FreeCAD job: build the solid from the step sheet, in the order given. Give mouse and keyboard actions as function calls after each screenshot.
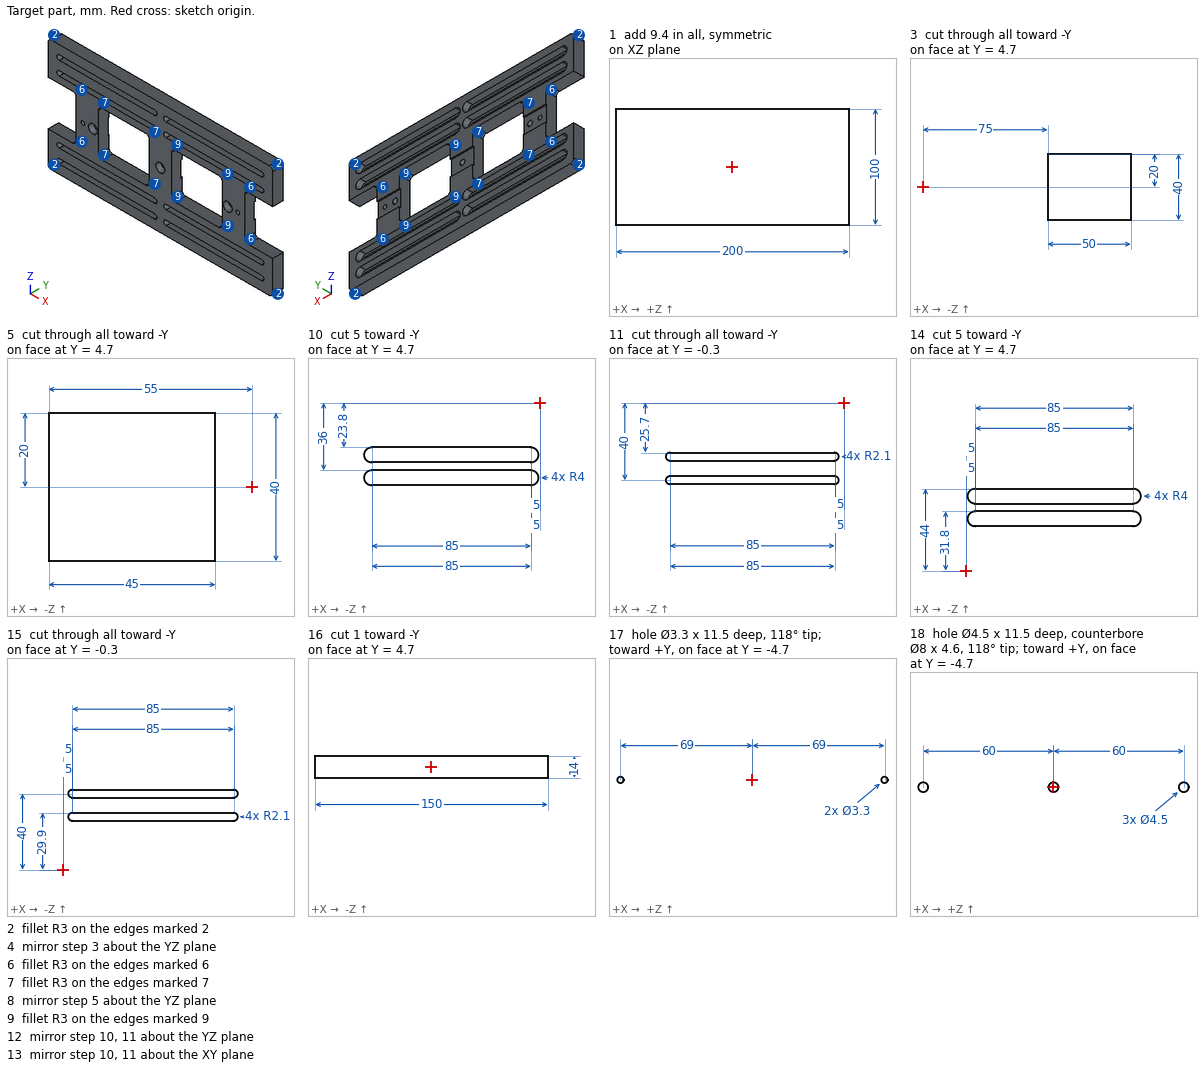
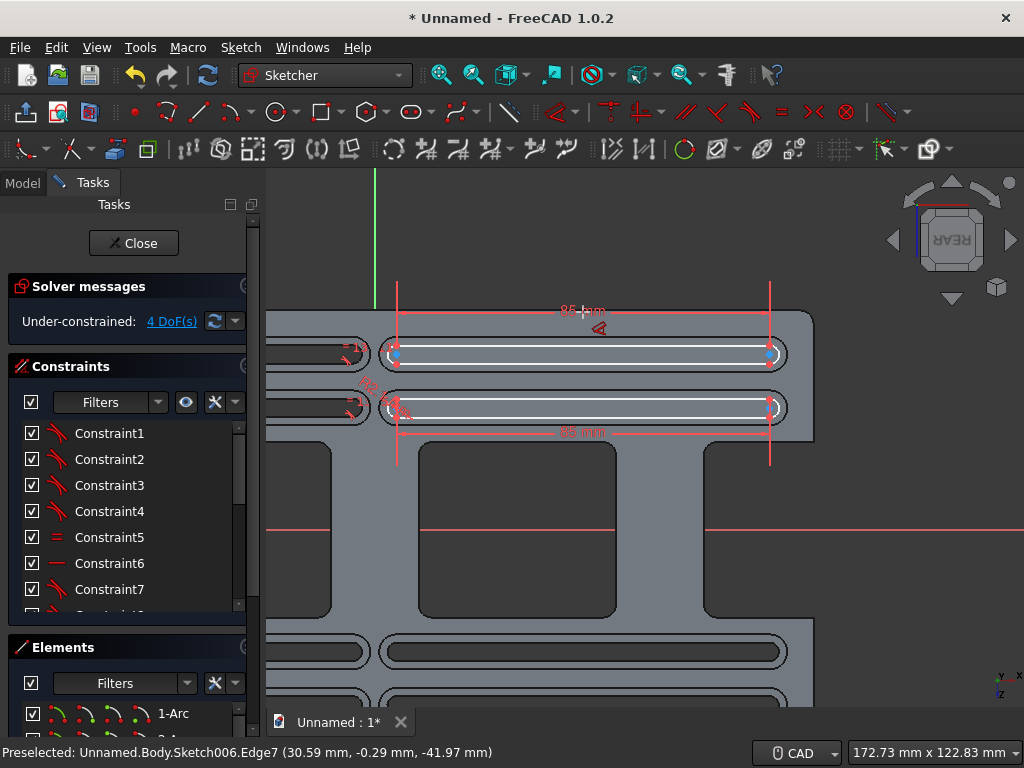
scroll(397, 399, up, 3)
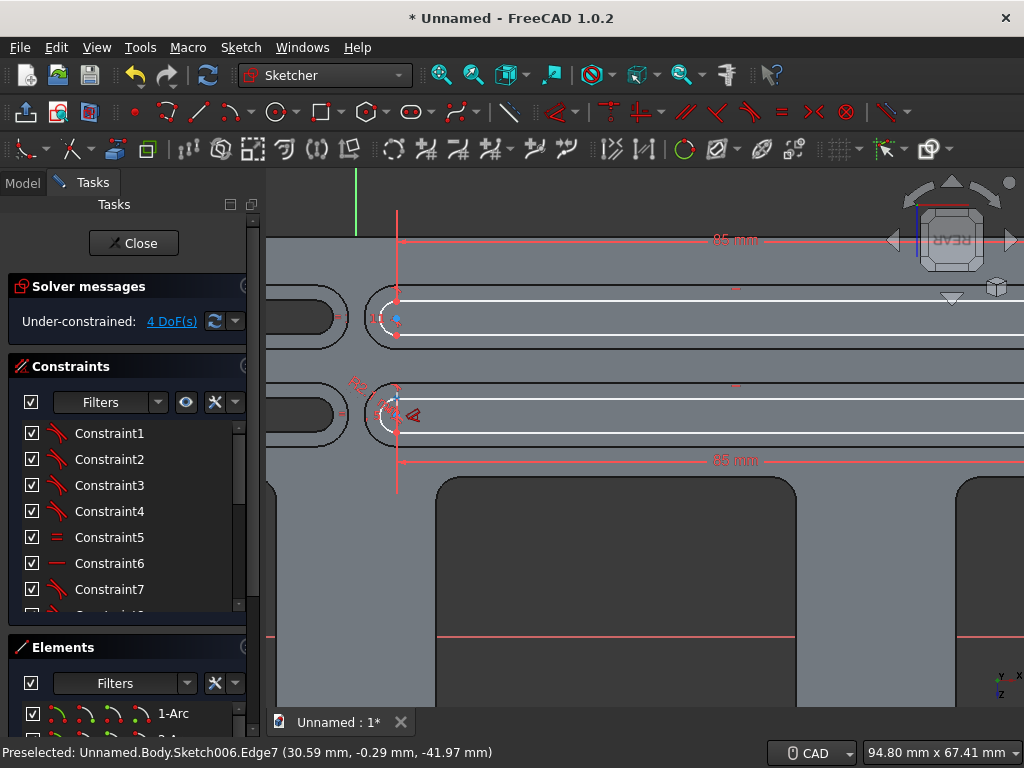
click(397, 399)
click(377, 671)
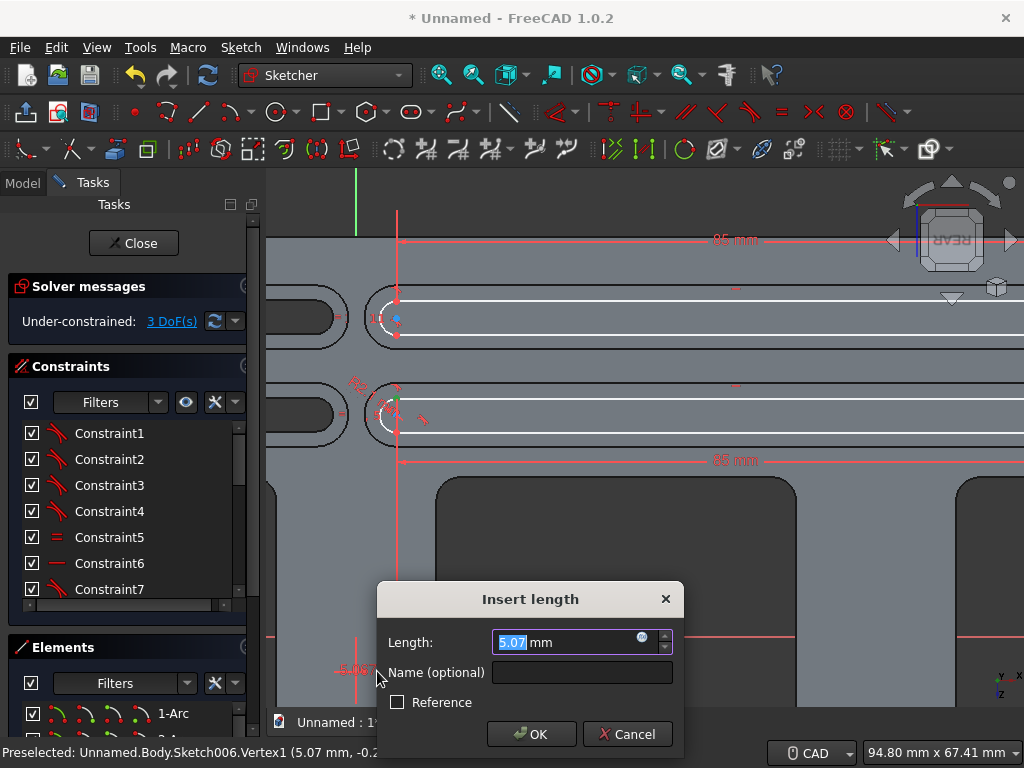
text(5)
key(Return)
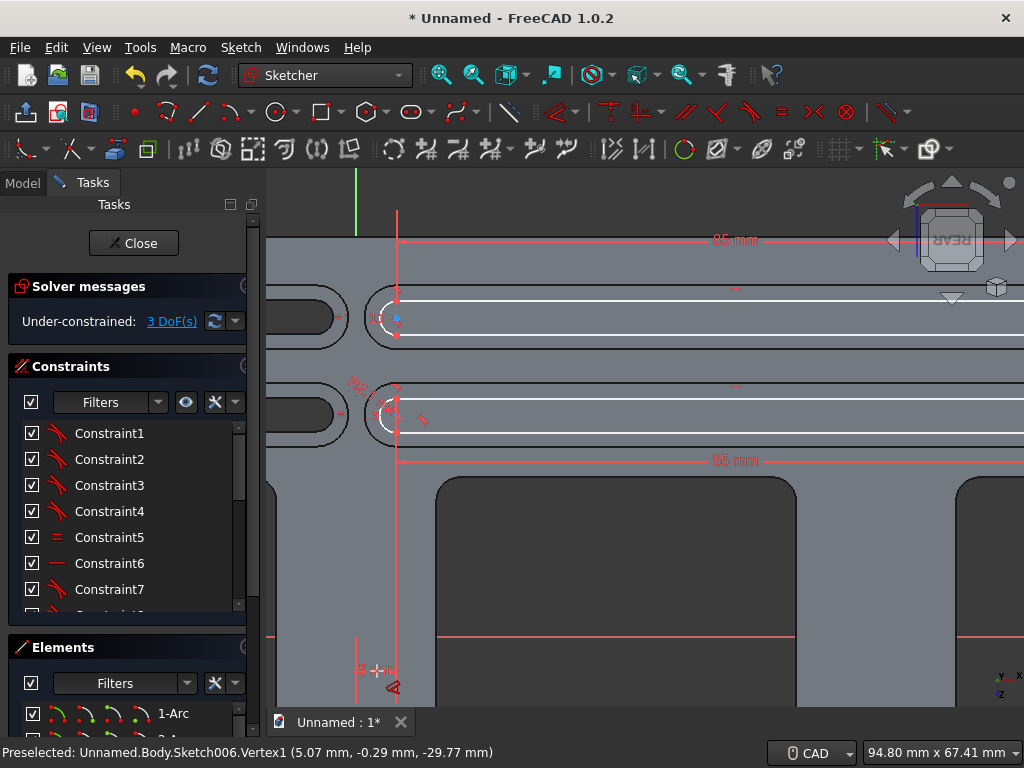
click(397, 301)
click(377, 267)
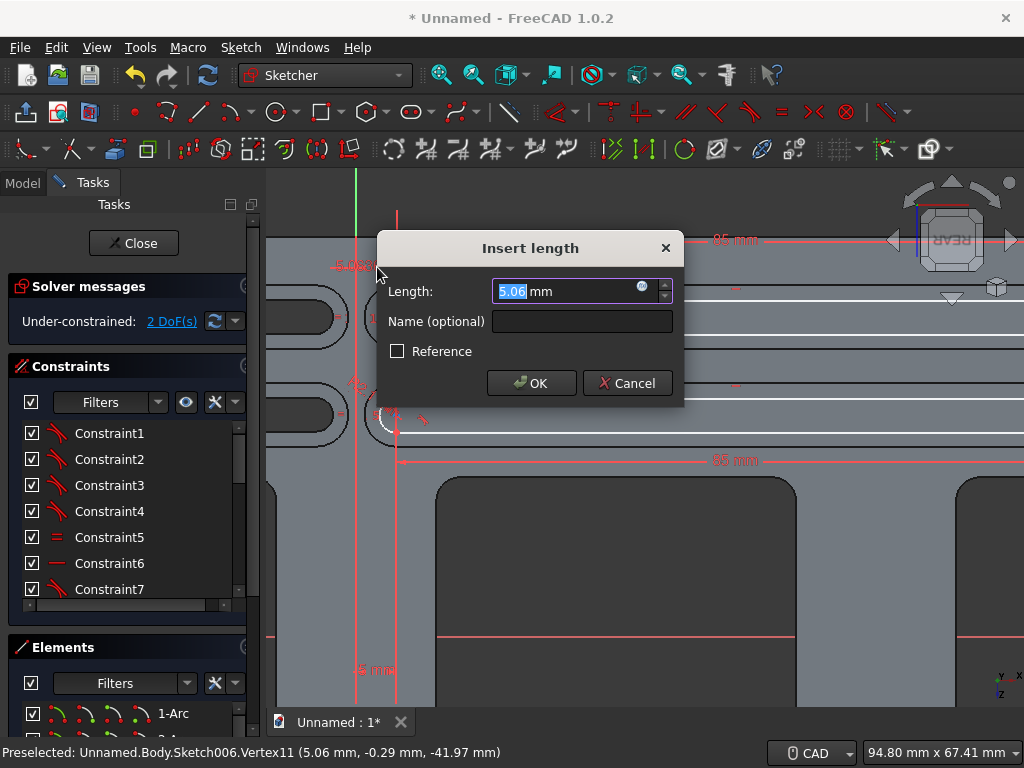
text(5)
key(Return)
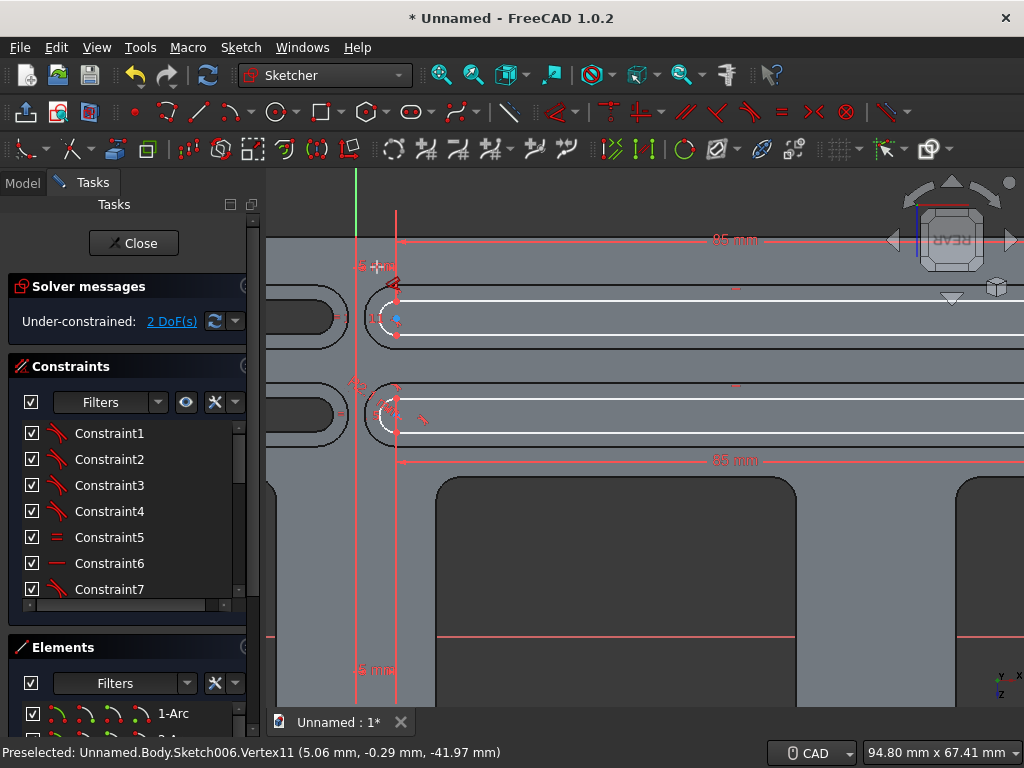
click(396, 318)
click(322, 478)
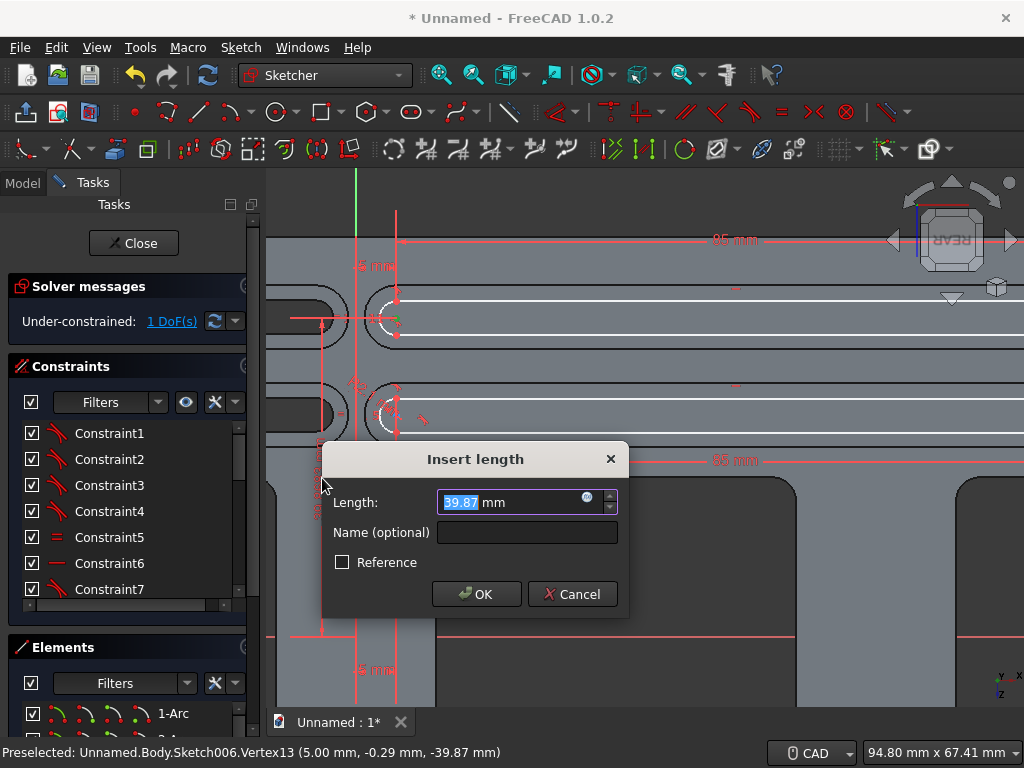
text(40)
key(Return)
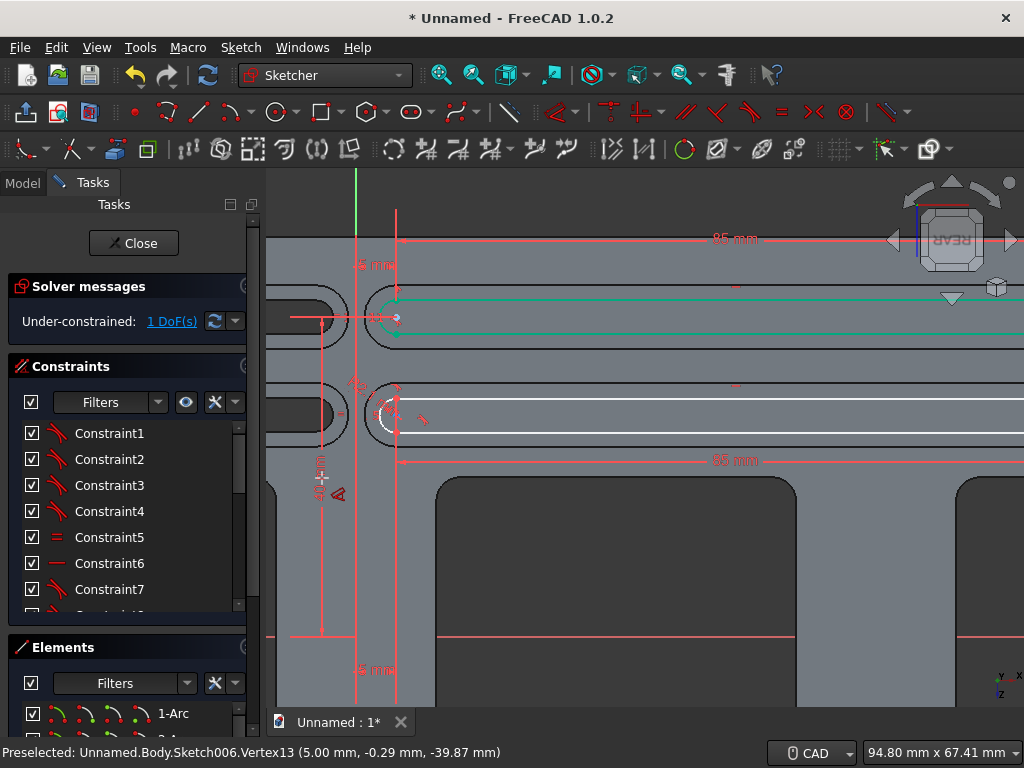
click(396, 399)
click(322, 518)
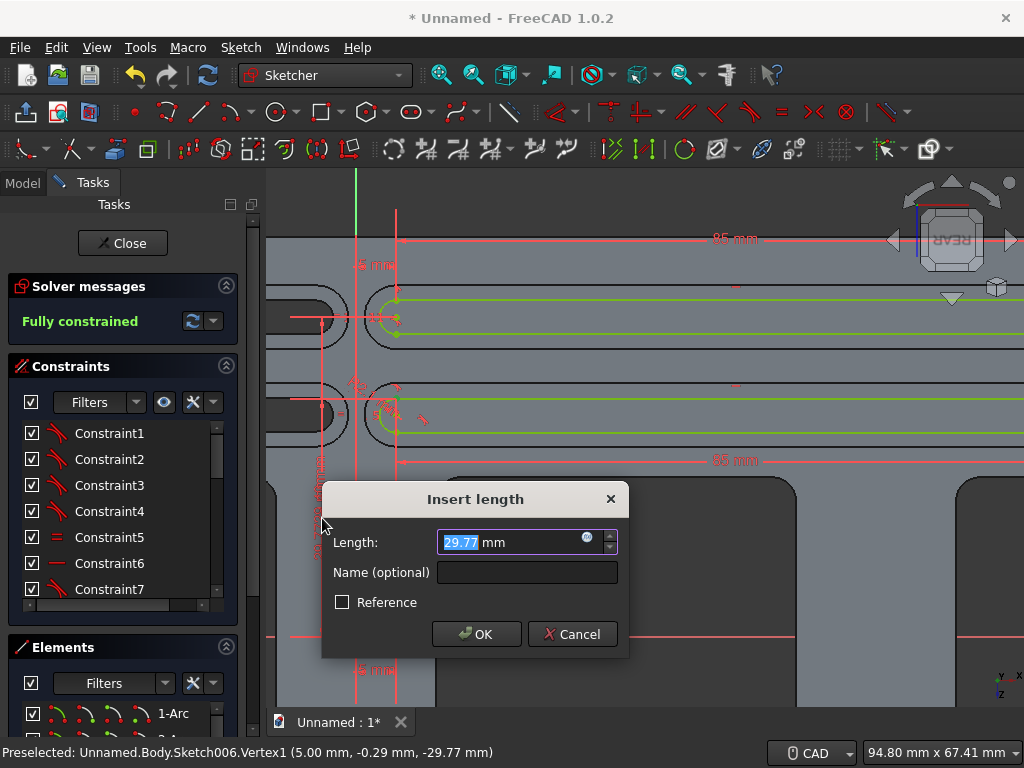
text(29.9)
key(Return)
key(Escape)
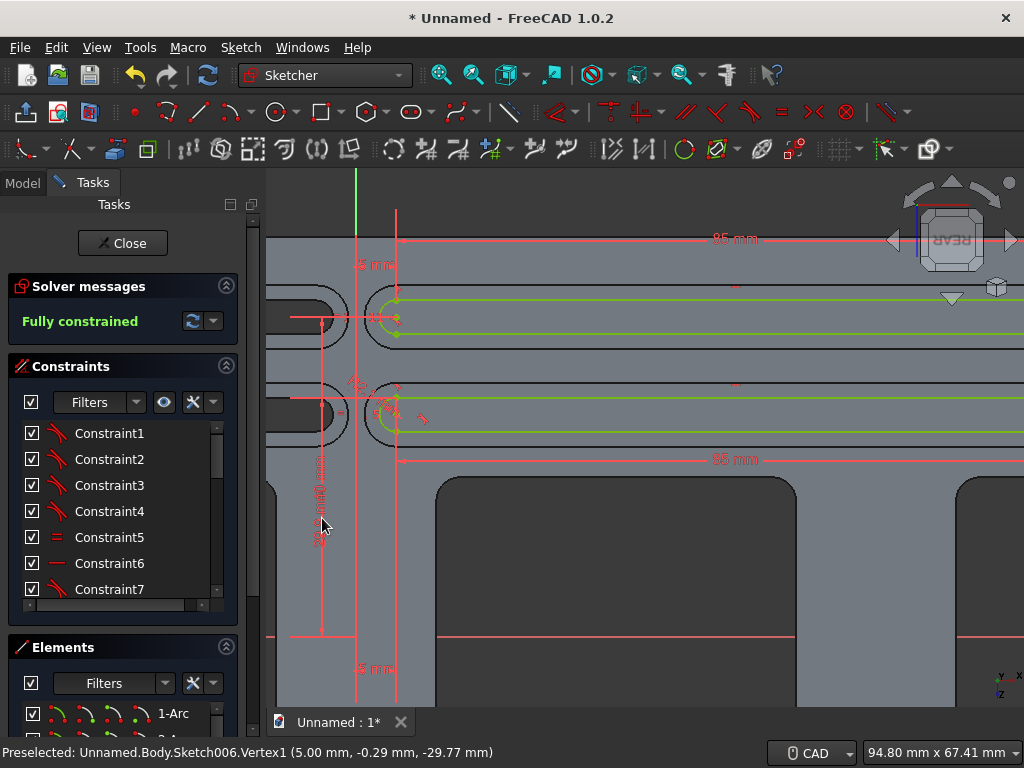
click(123, 243)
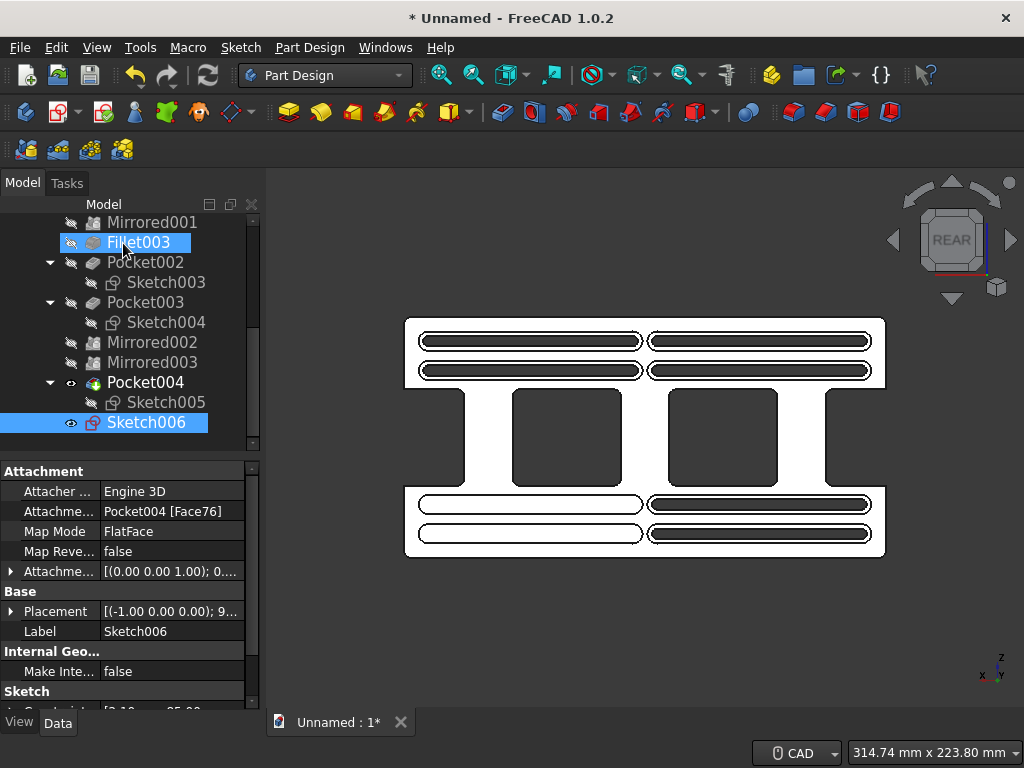
click(504, 112)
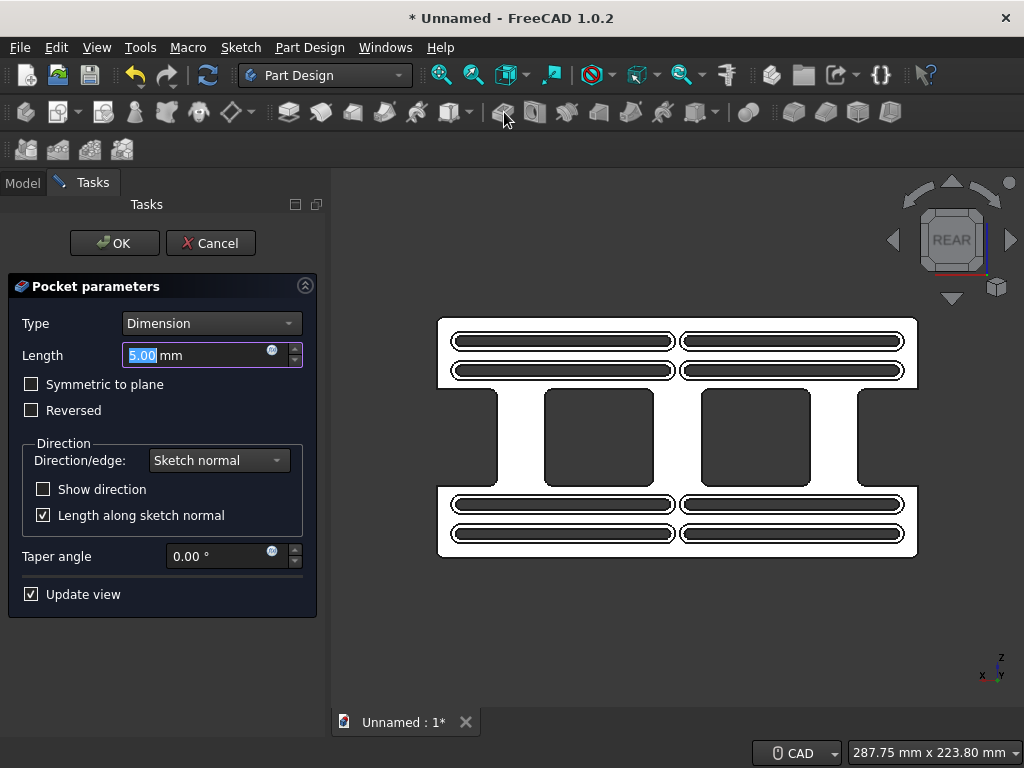
click(212, 324)